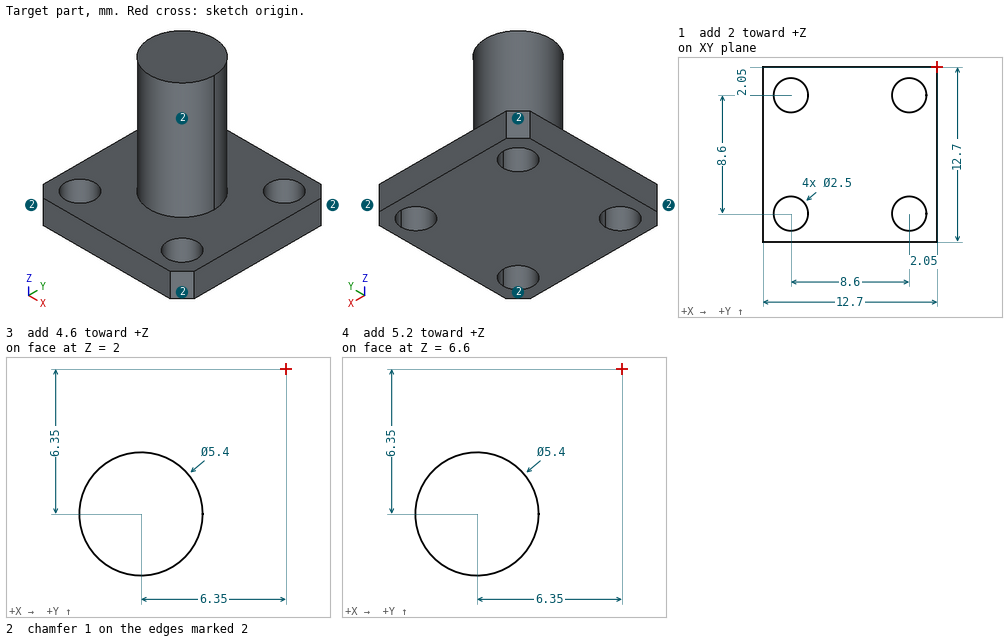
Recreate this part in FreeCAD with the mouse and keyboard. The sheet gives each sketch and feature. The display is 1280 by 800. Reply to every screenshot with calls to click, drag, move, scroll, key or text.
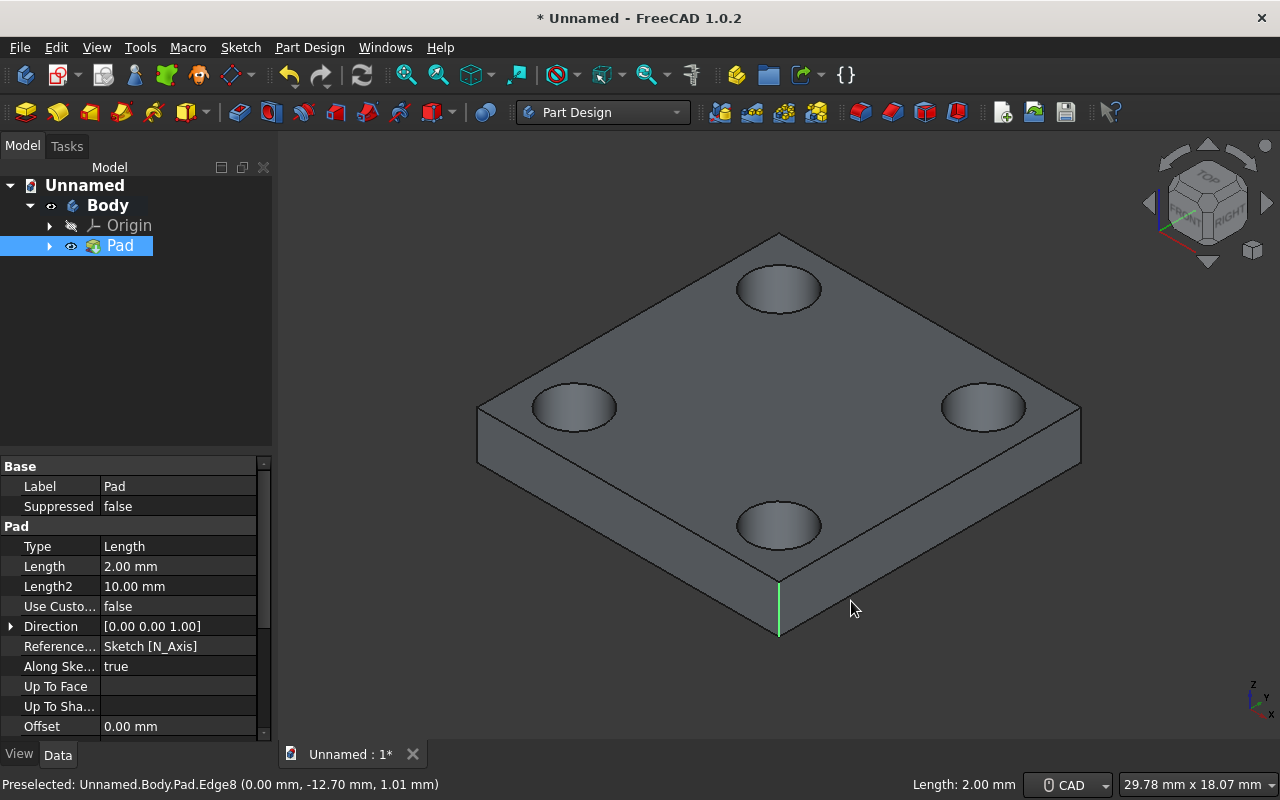
key(2)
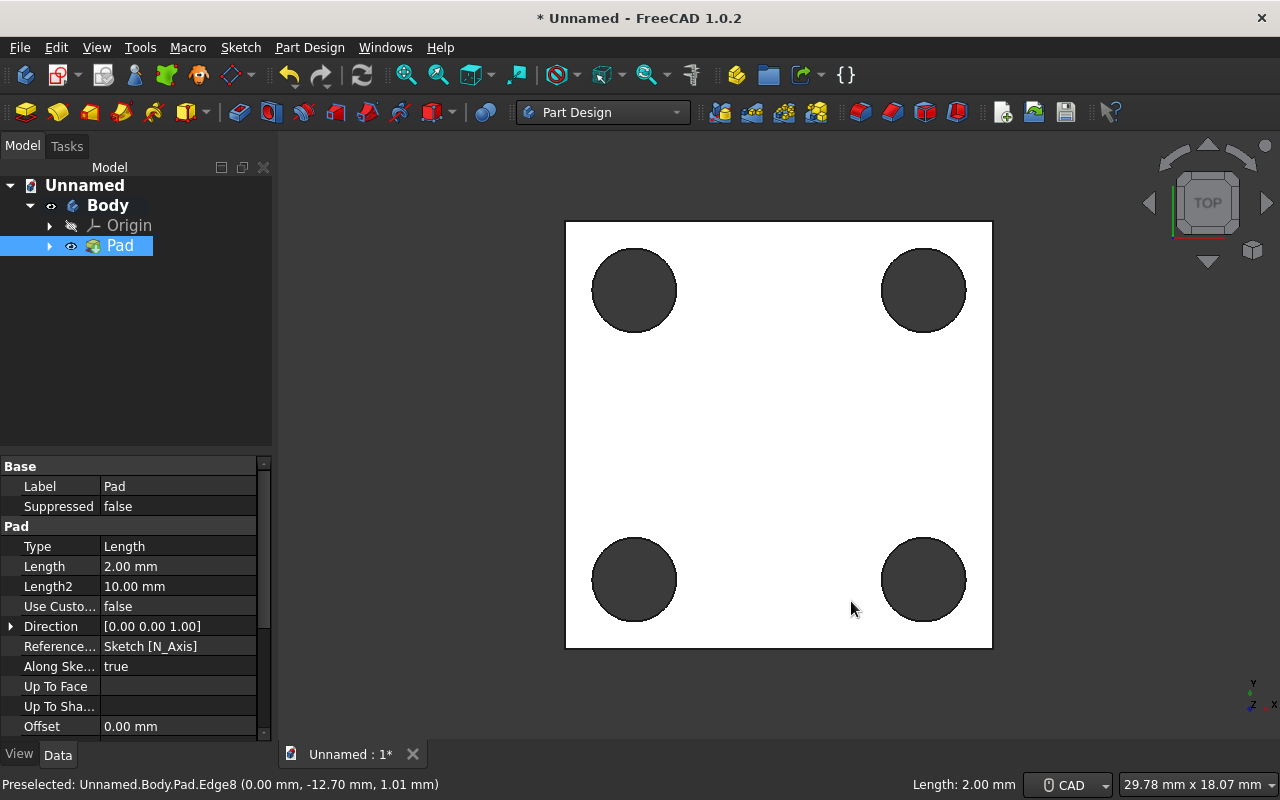
key(1)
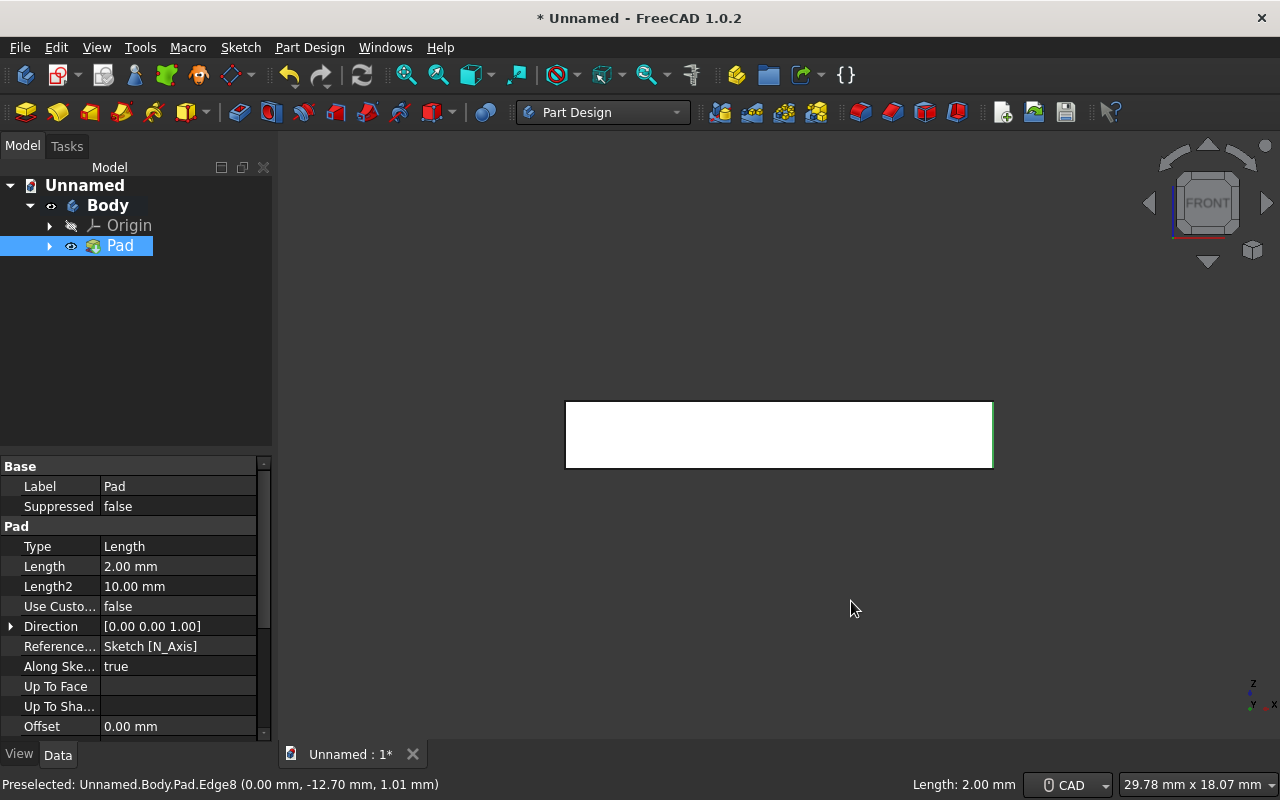
click(408, 76)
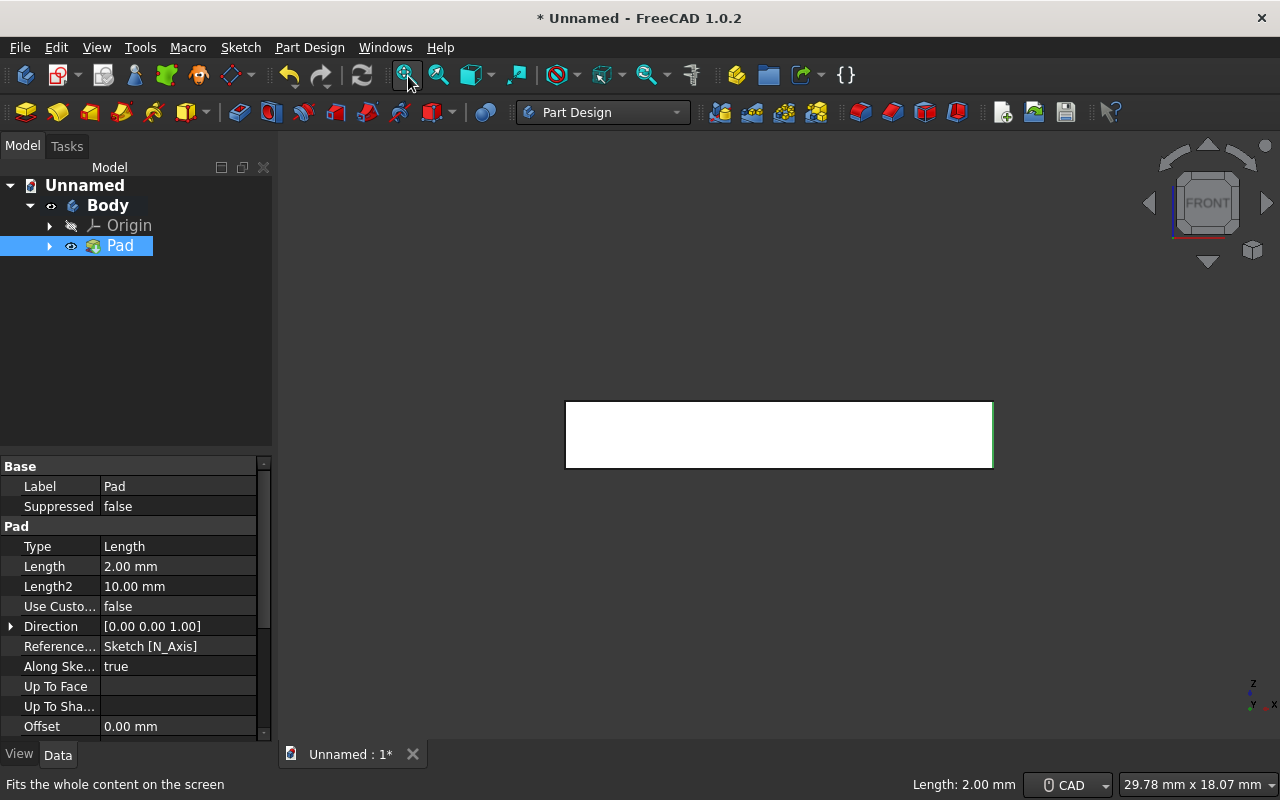
click(565, 434, ctrl)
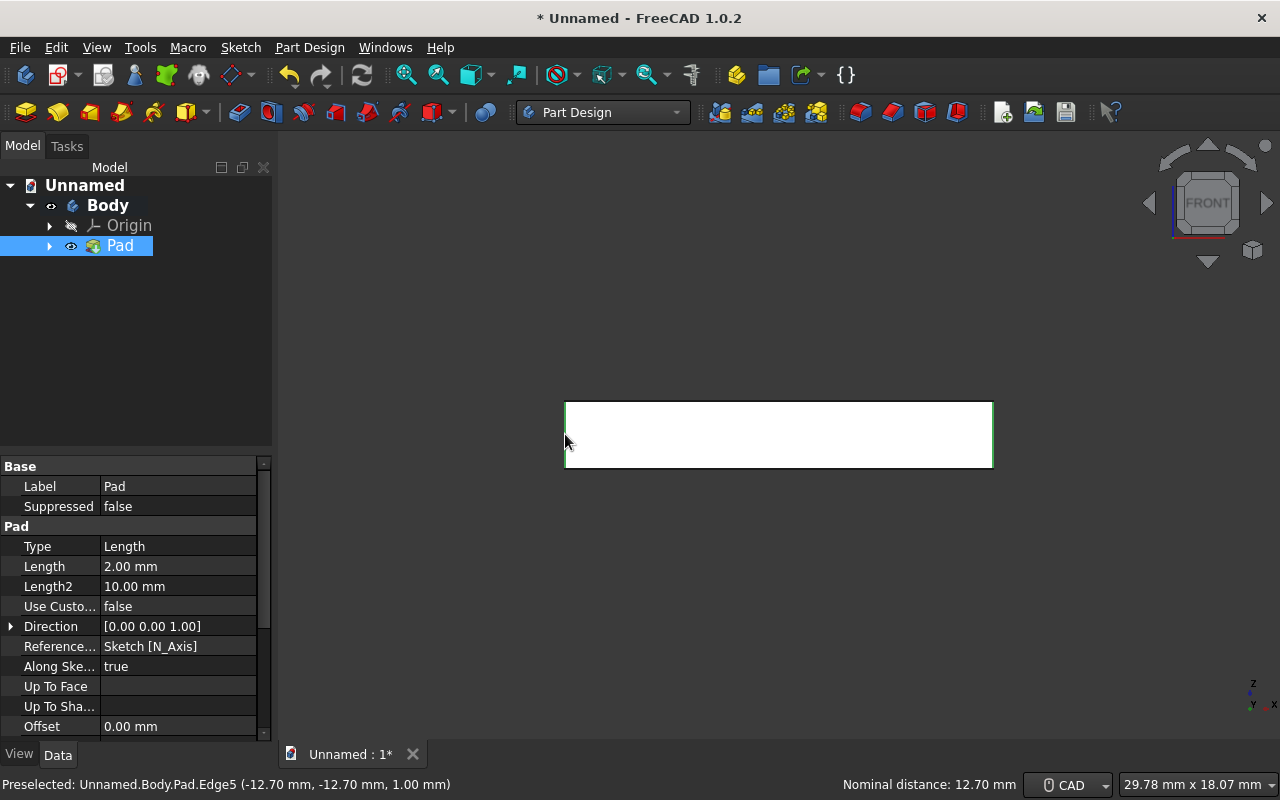
key(3)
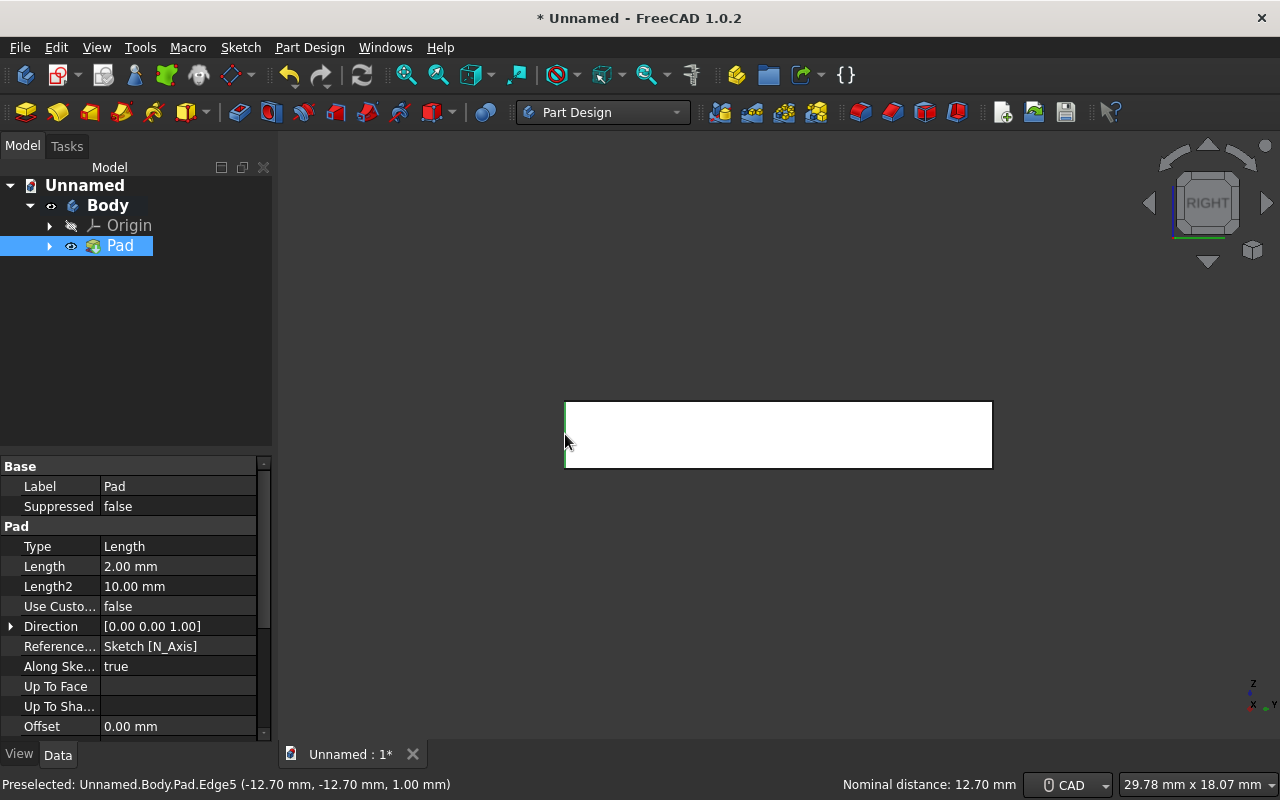
click(408, 76)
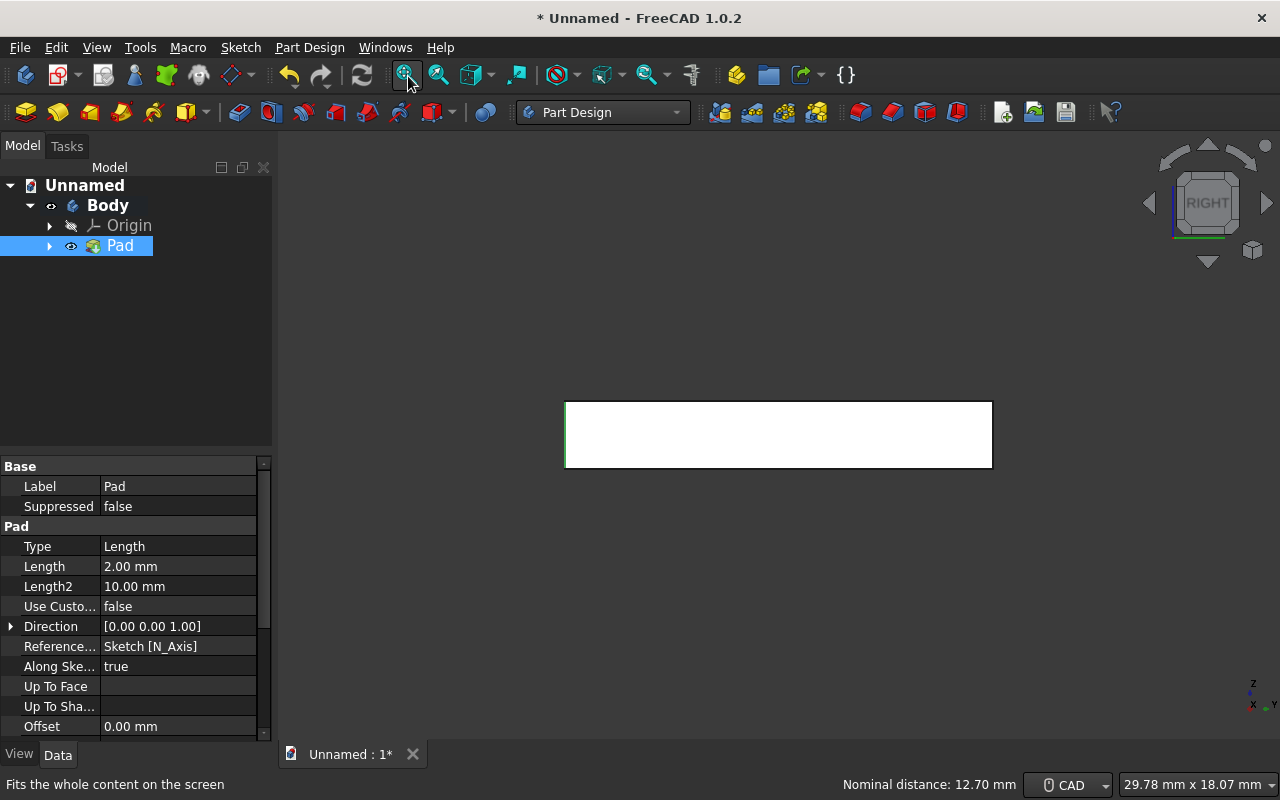
click(993, 434, ctrl)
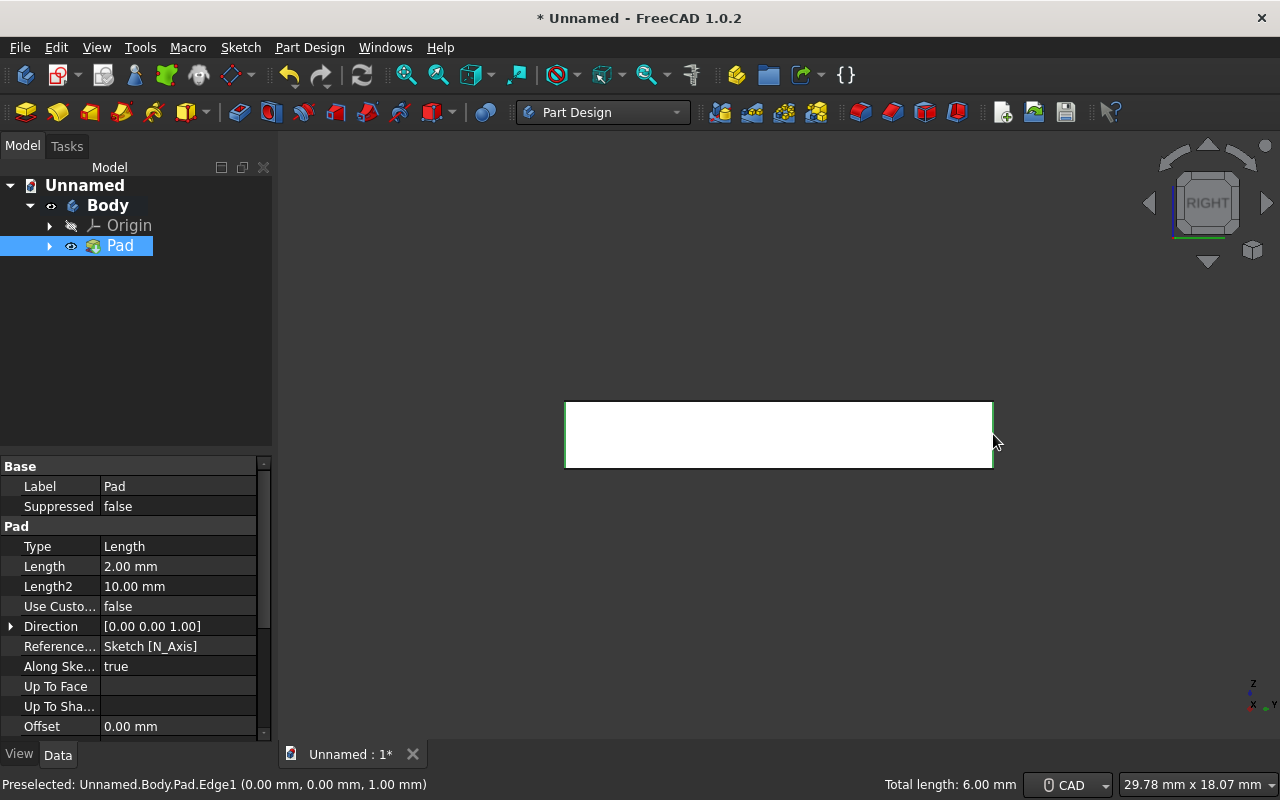
key(5)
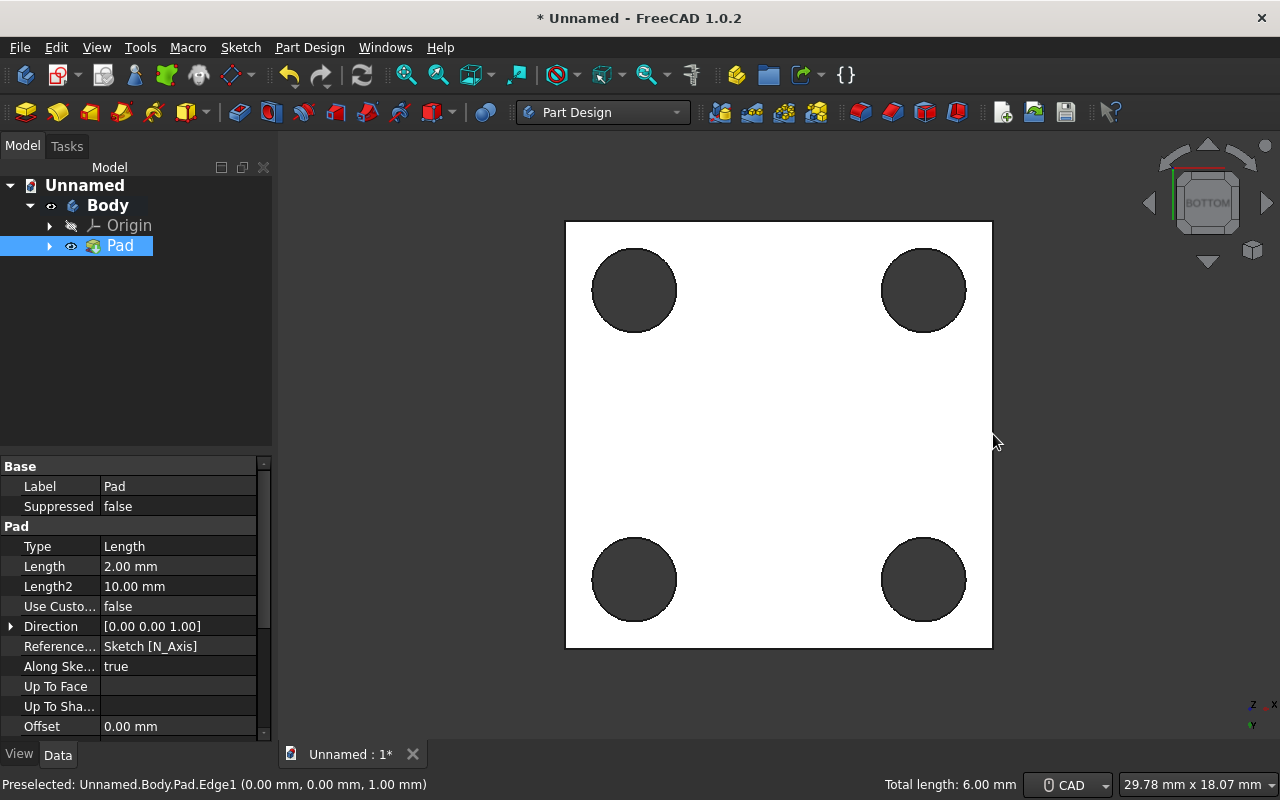
key(4)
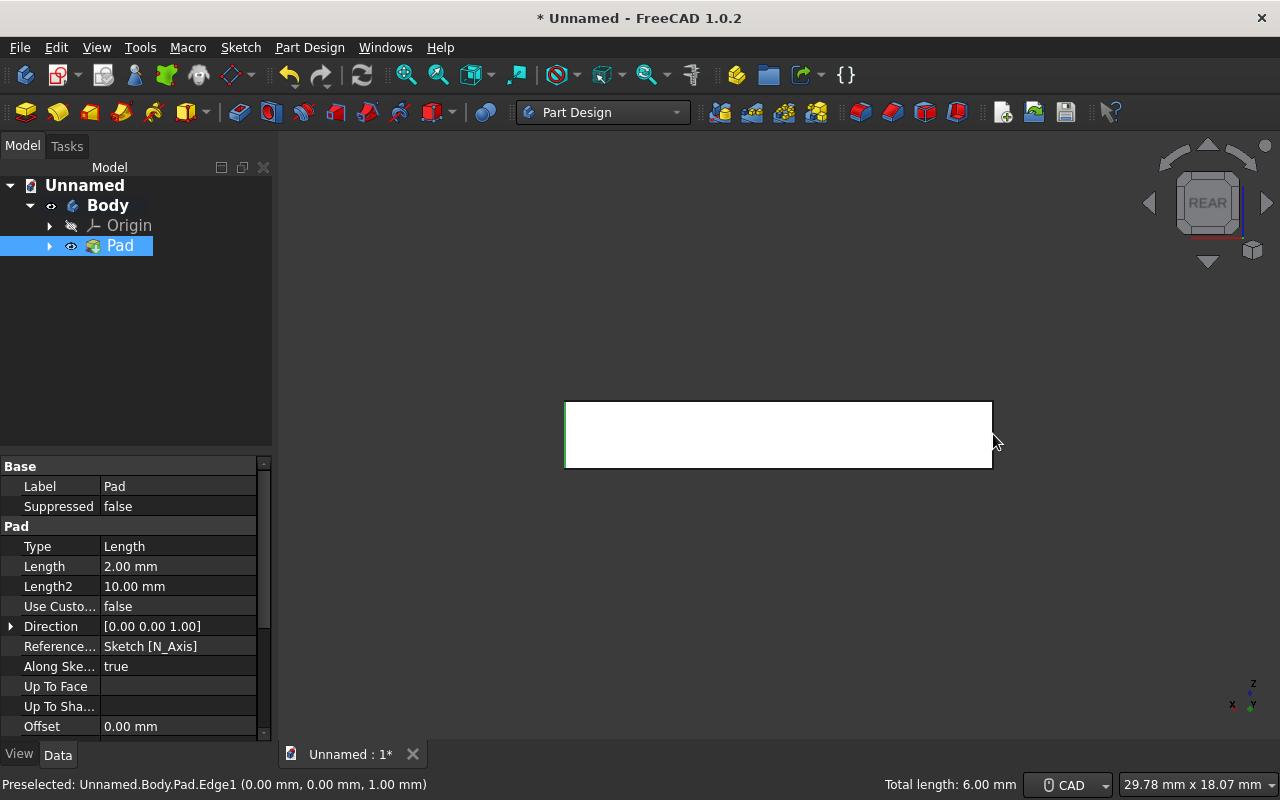
click(408, 76)